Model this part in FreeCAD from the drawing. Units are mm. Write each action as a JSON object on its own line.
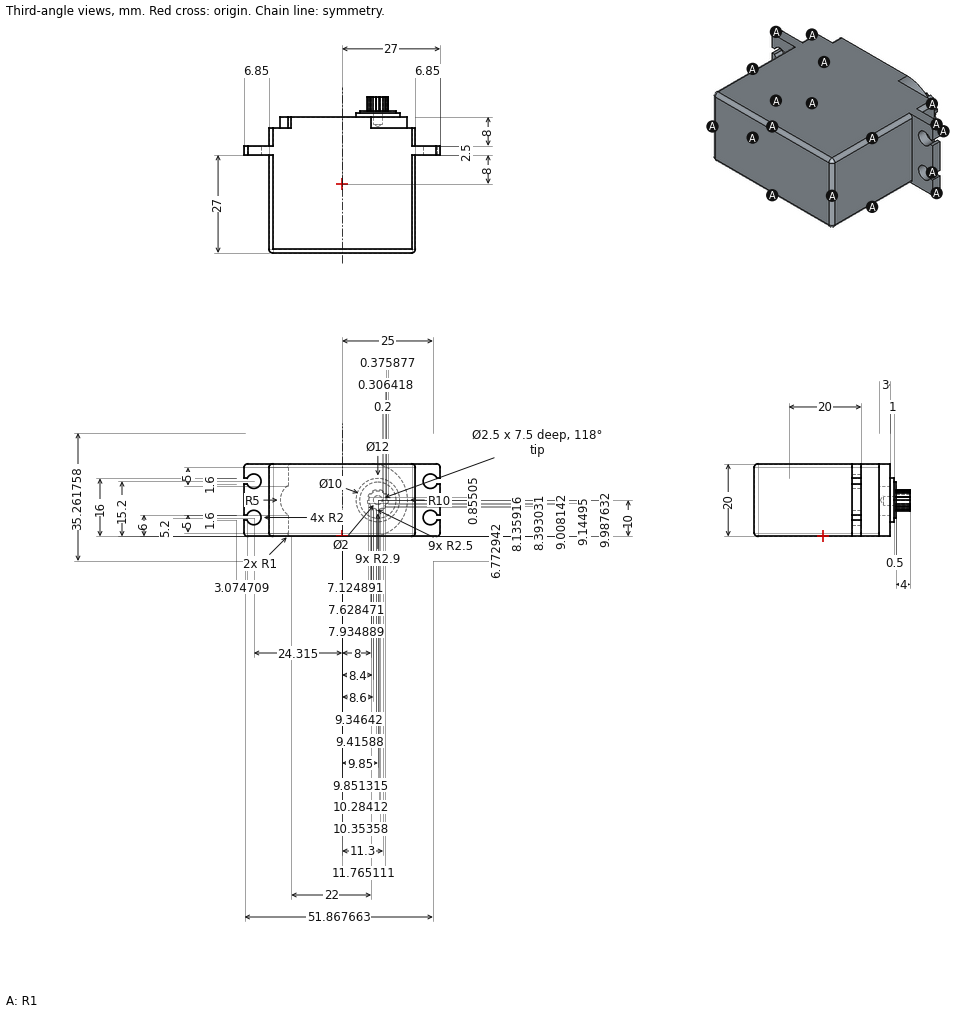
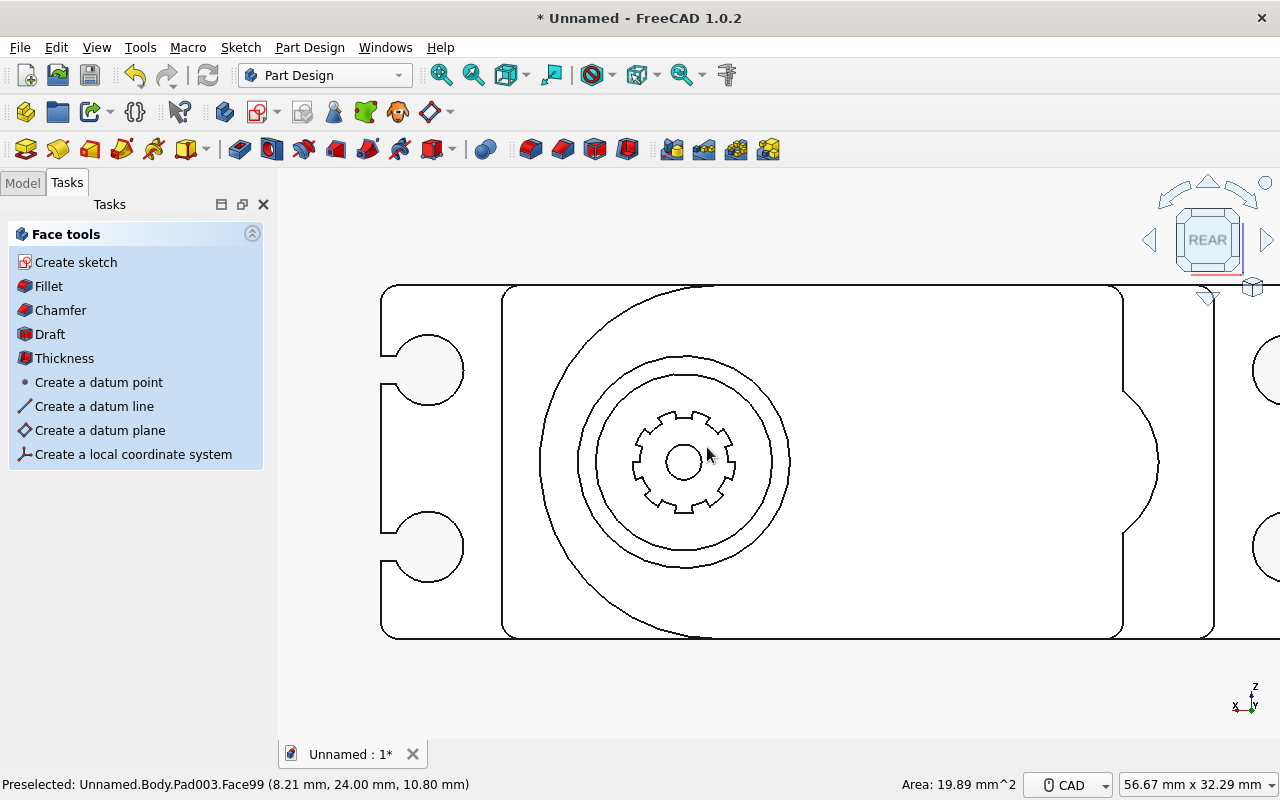
{"action": "left_click", "coordinate": [258, 112]}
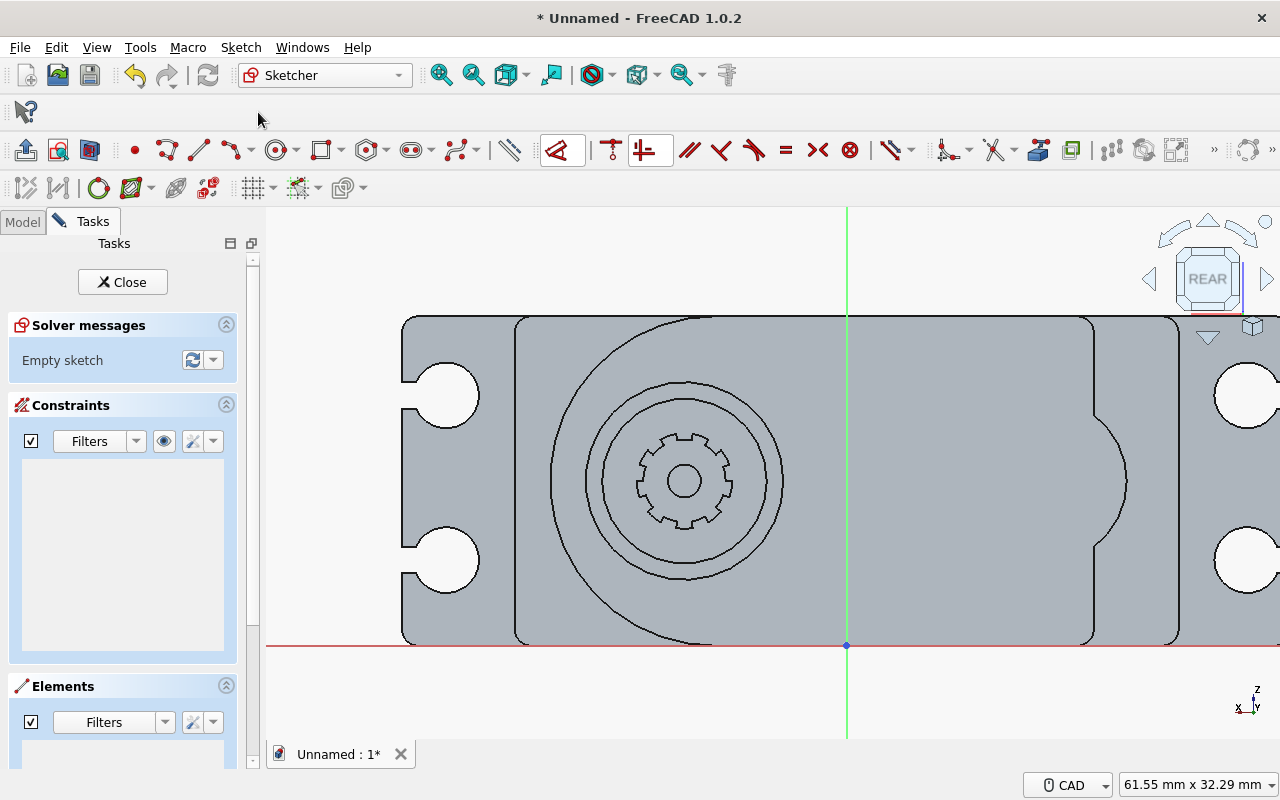
{"action": "scroll", "coordinate": [681, 482], "scroll_direction": "up", "scroll_amount": 10}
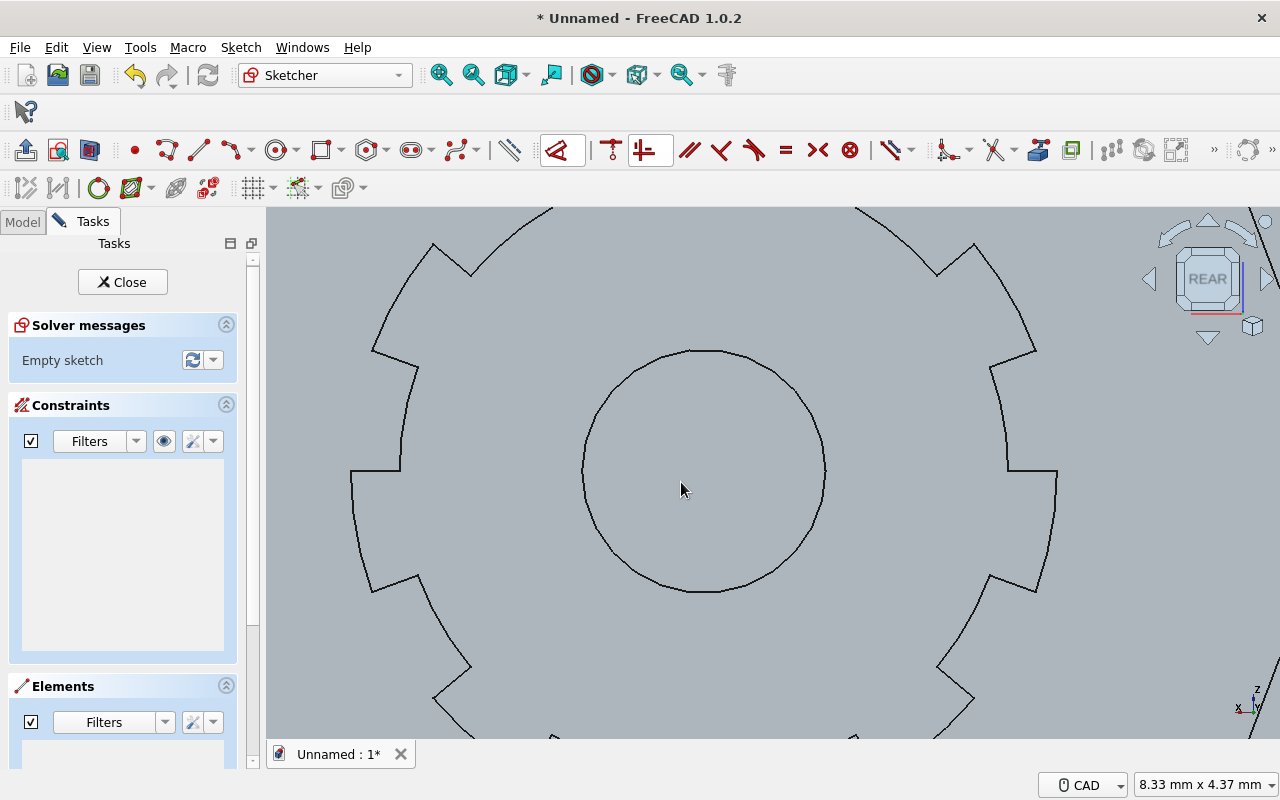
{"action": "left_click", "coordinate": [276, 150]}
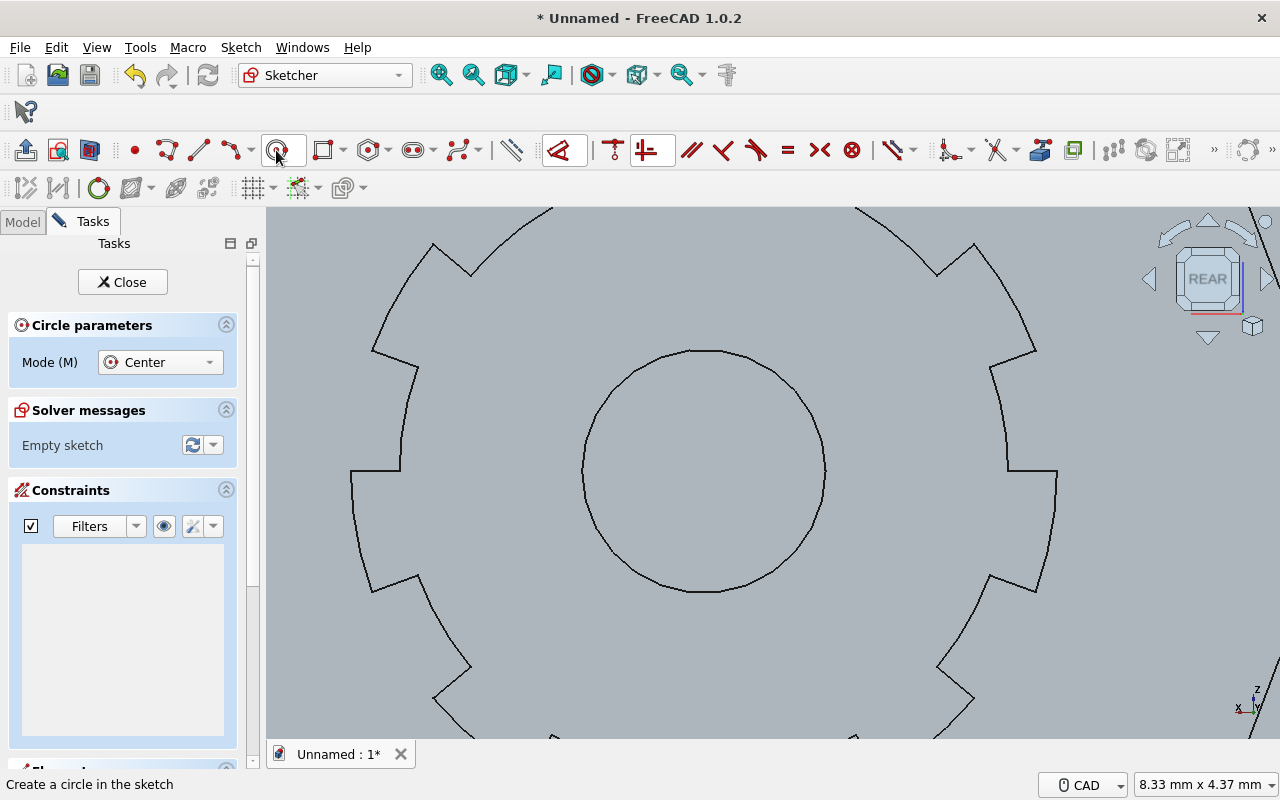
{"action": "left_click", "coordinate": [704, 471]}
{"action": "mouse_move", "coordinate": [811, 364]}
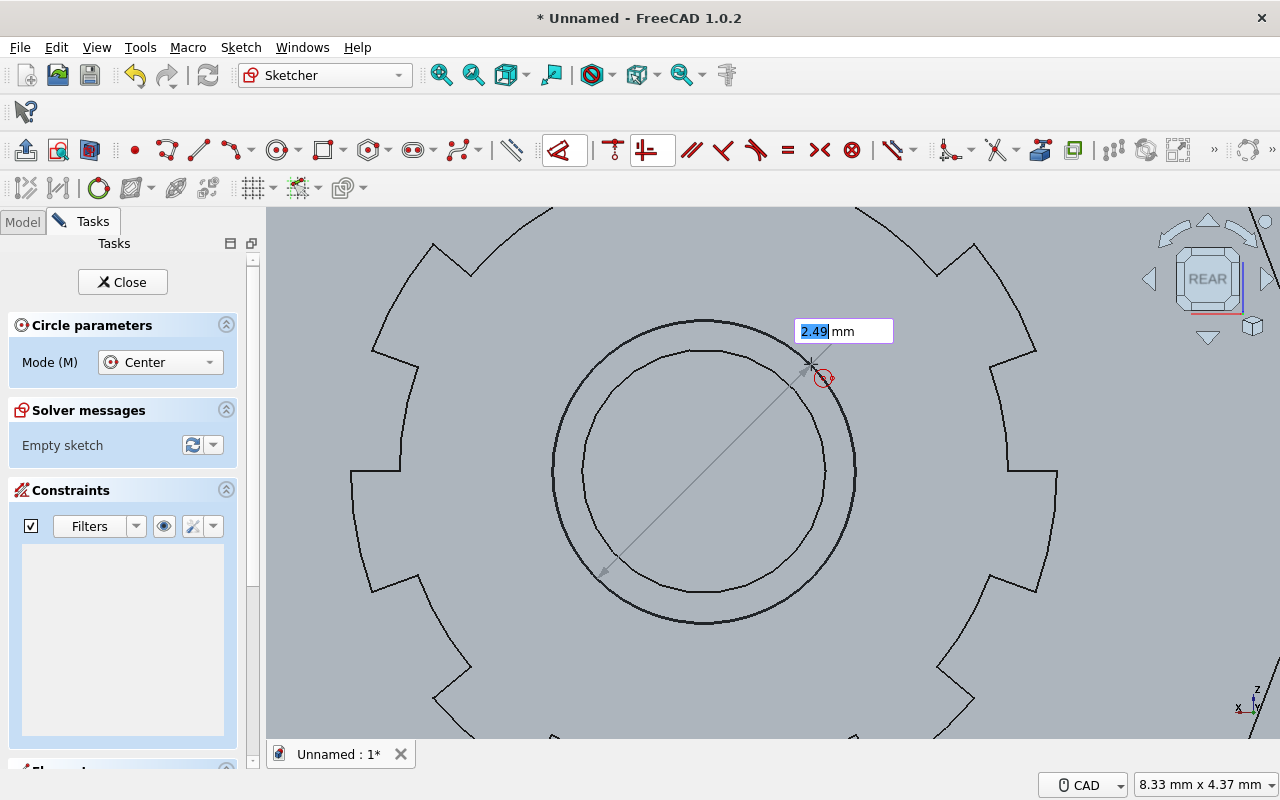
{"action": "type", "text": "2.5"}
{"action": "key", "text": "Return"}
{"action": "key", "text": "Escape"}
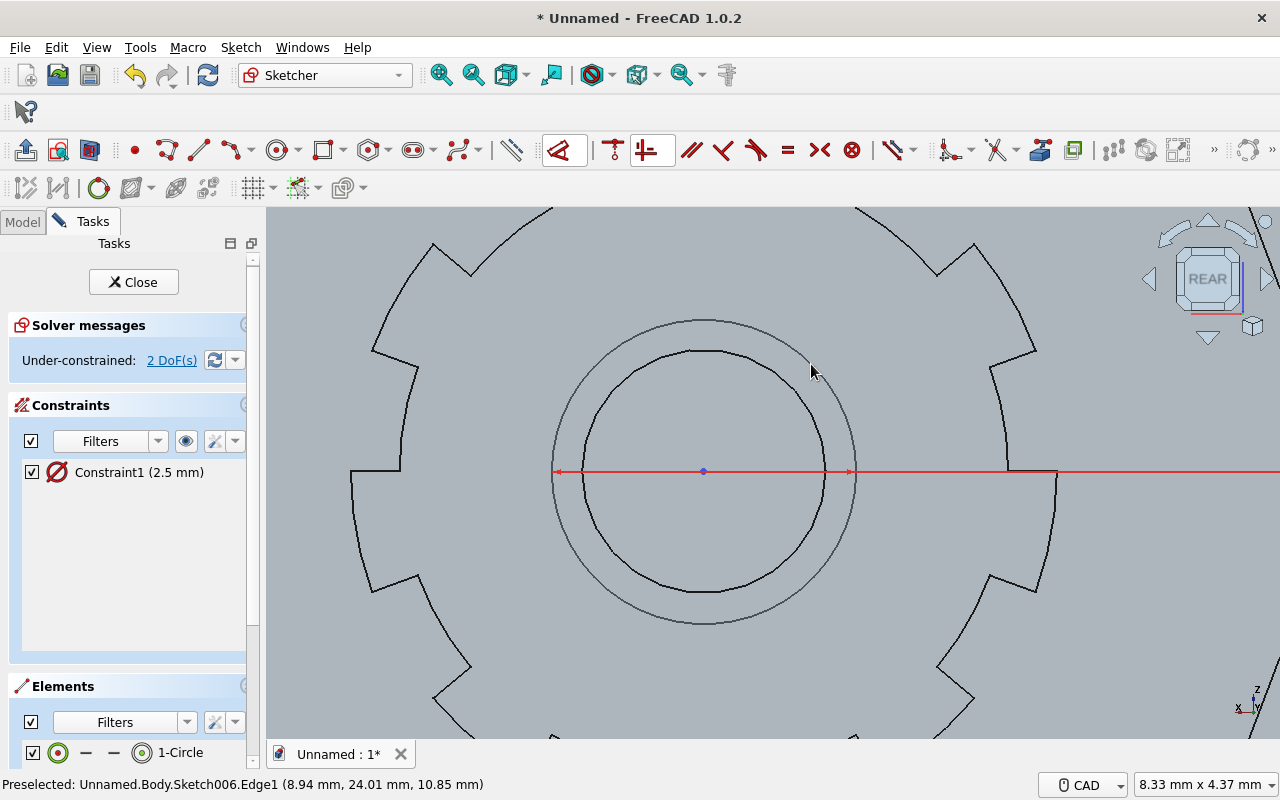
{"action": "left_click", "coordinate": [704, 472]}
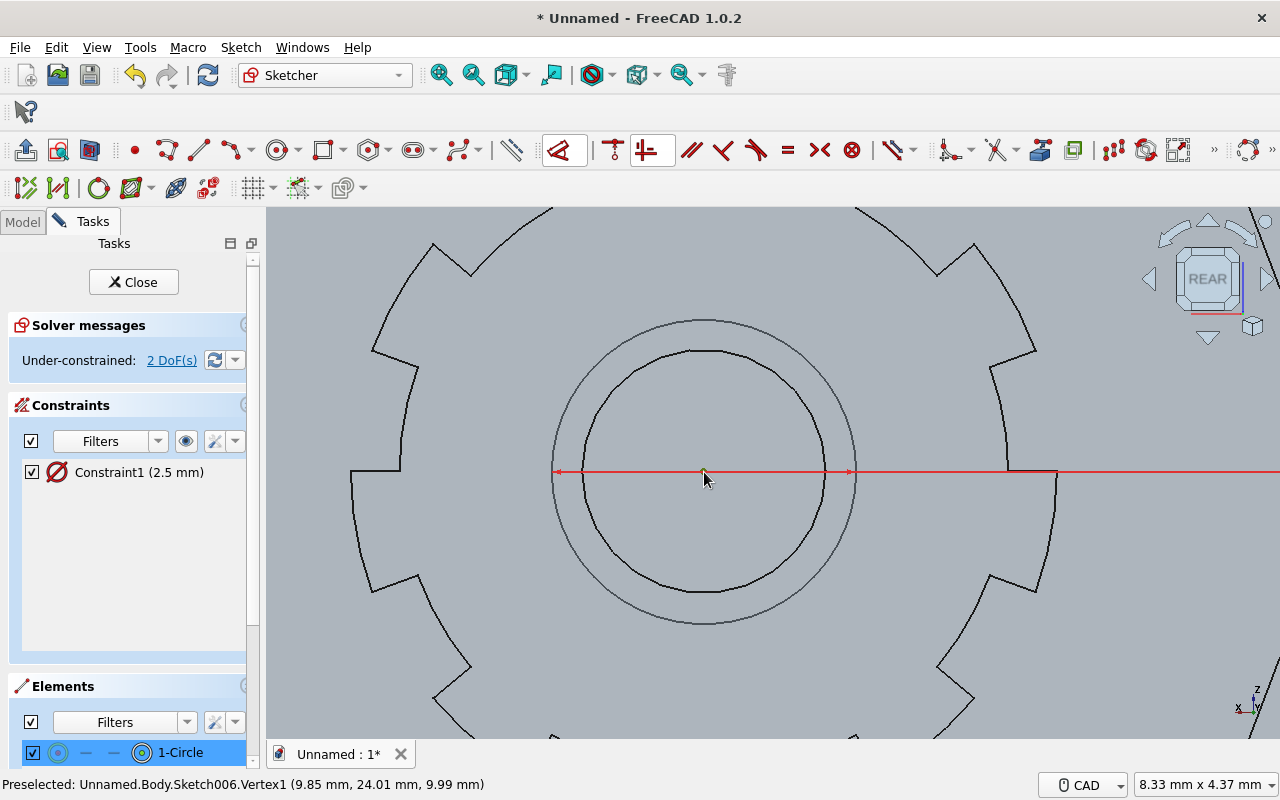
{"action": "left_click", "coordinate": [582, 150]}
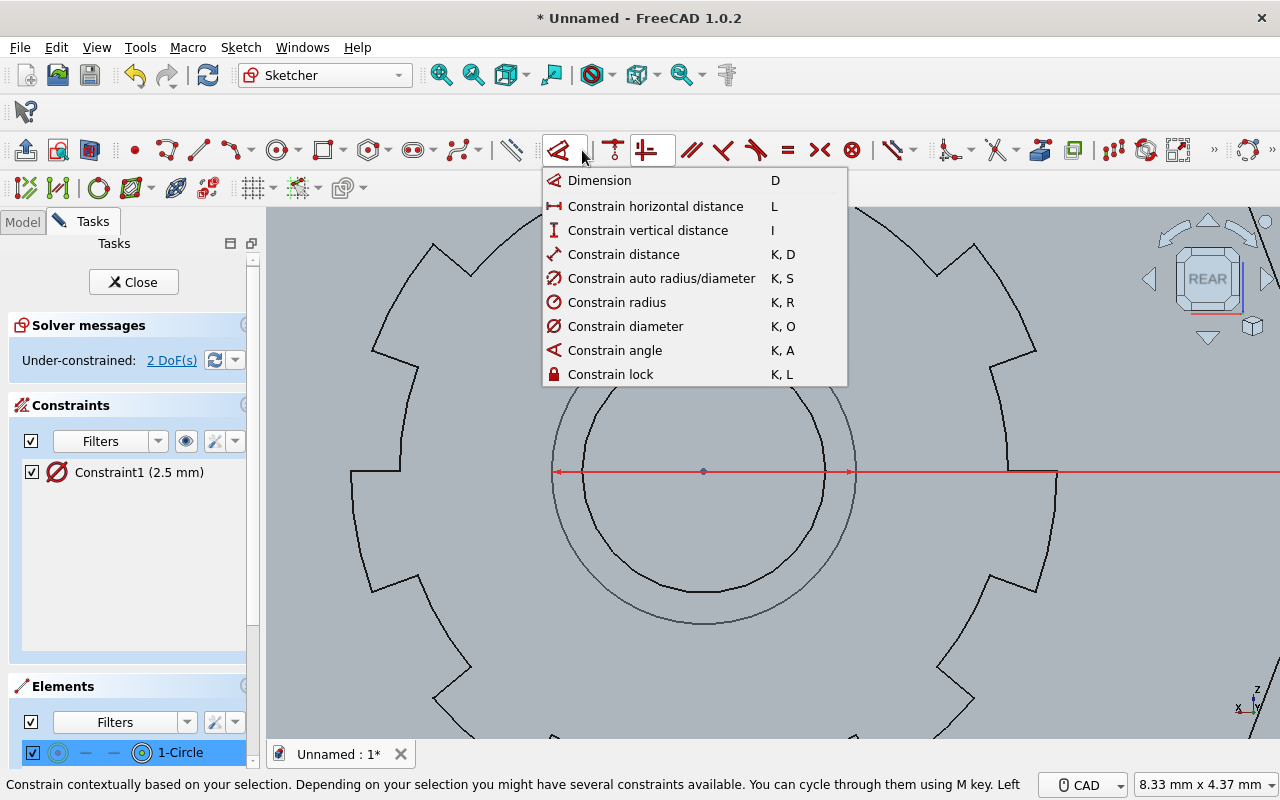
{"action": "left_click", "coordinate": [695, 230]}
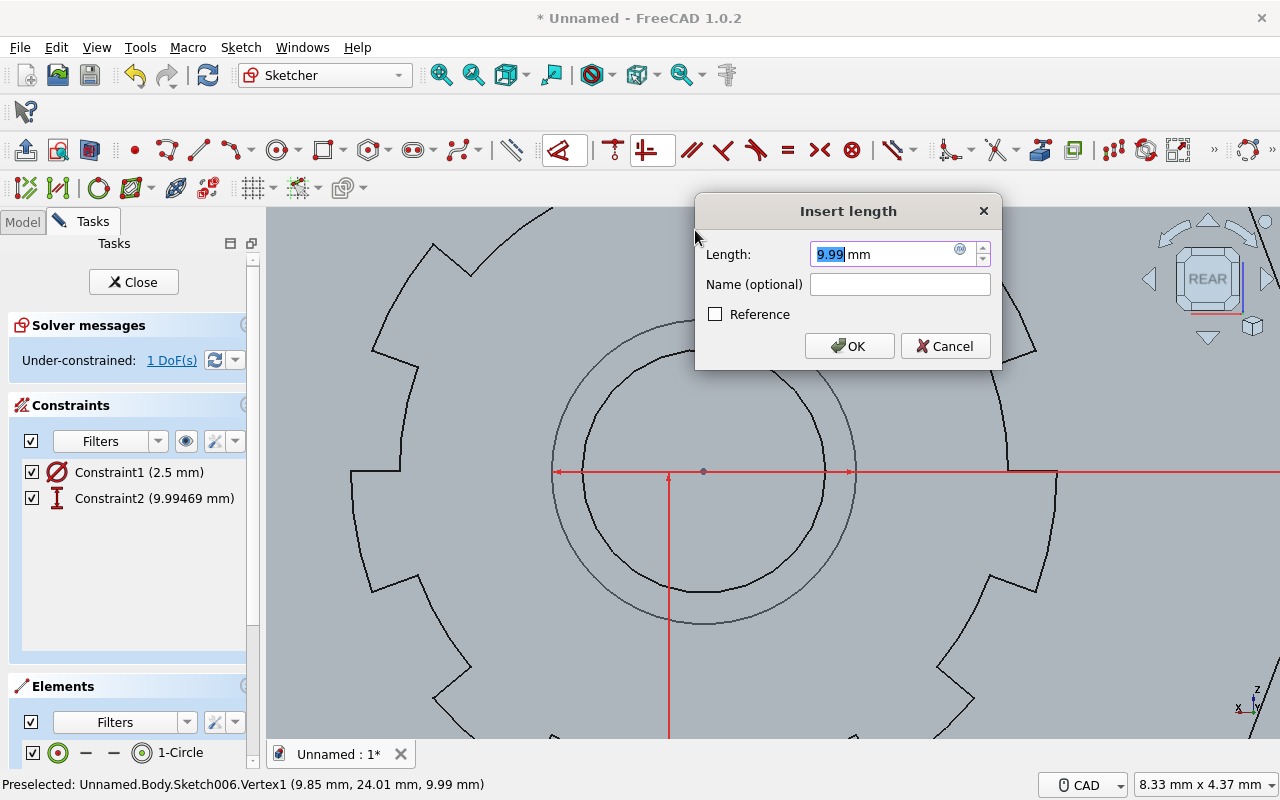
{"action": "type", "text": "10"}
{"action": "key", "text": "Return"}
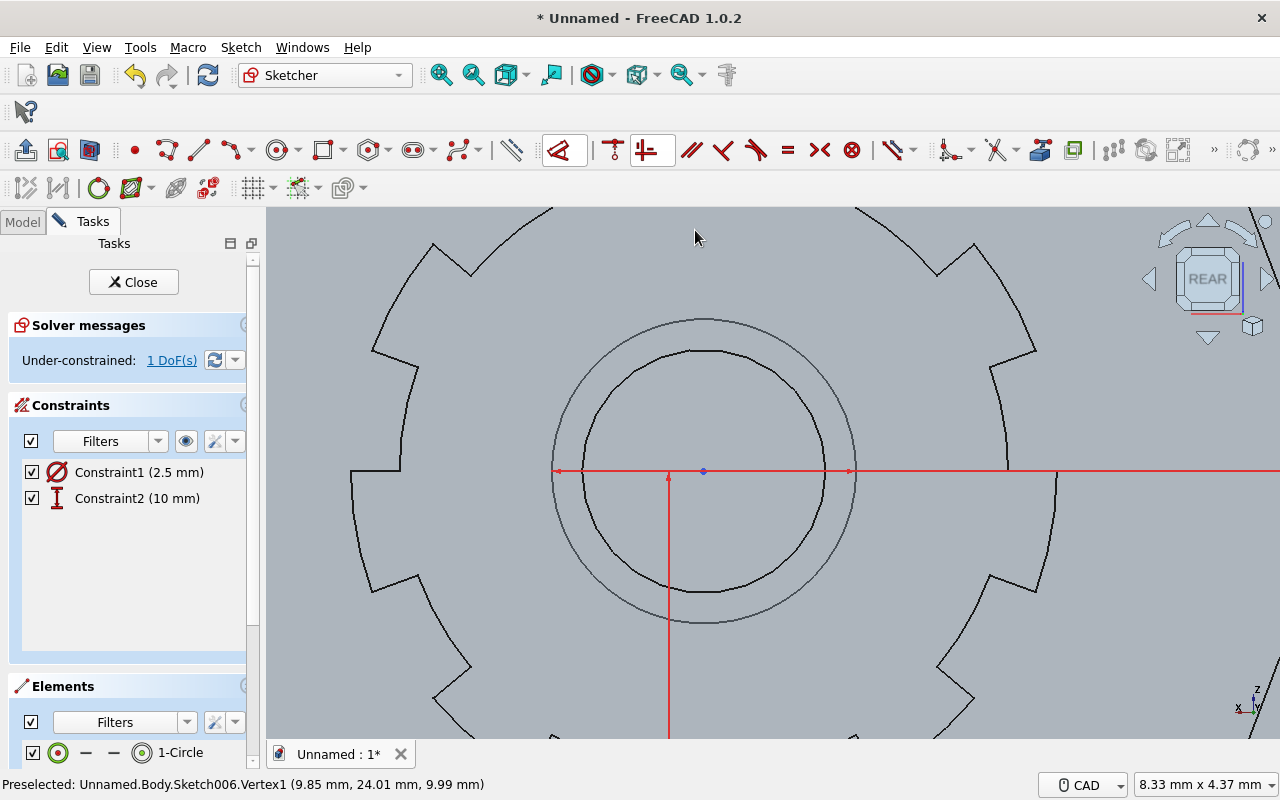
{"action": "left_click", "coordinate": [704, 471]}